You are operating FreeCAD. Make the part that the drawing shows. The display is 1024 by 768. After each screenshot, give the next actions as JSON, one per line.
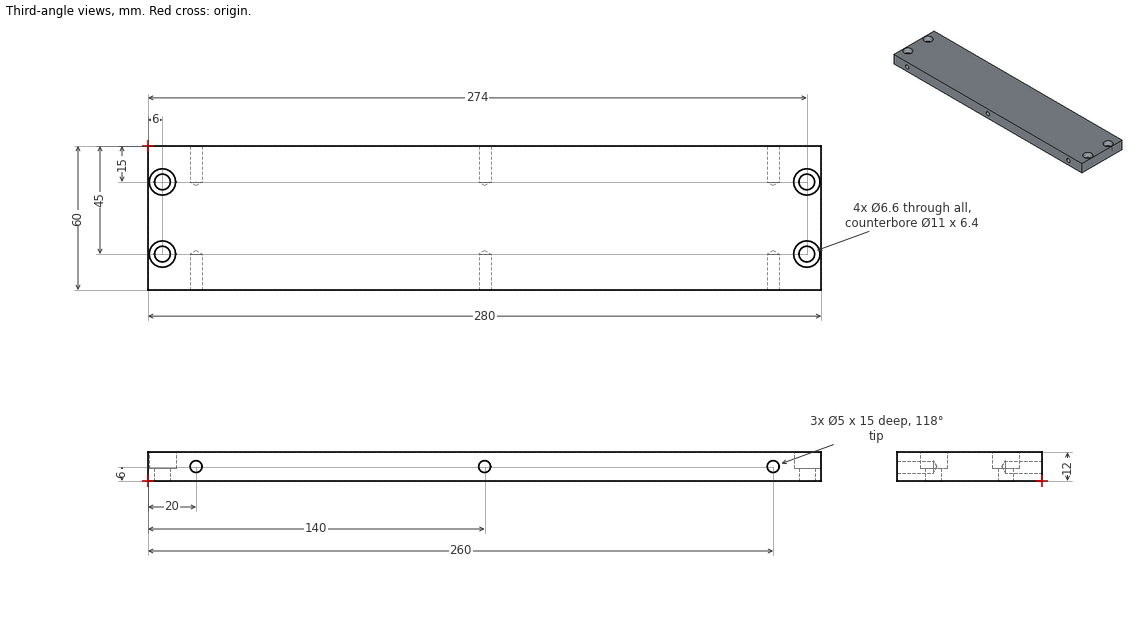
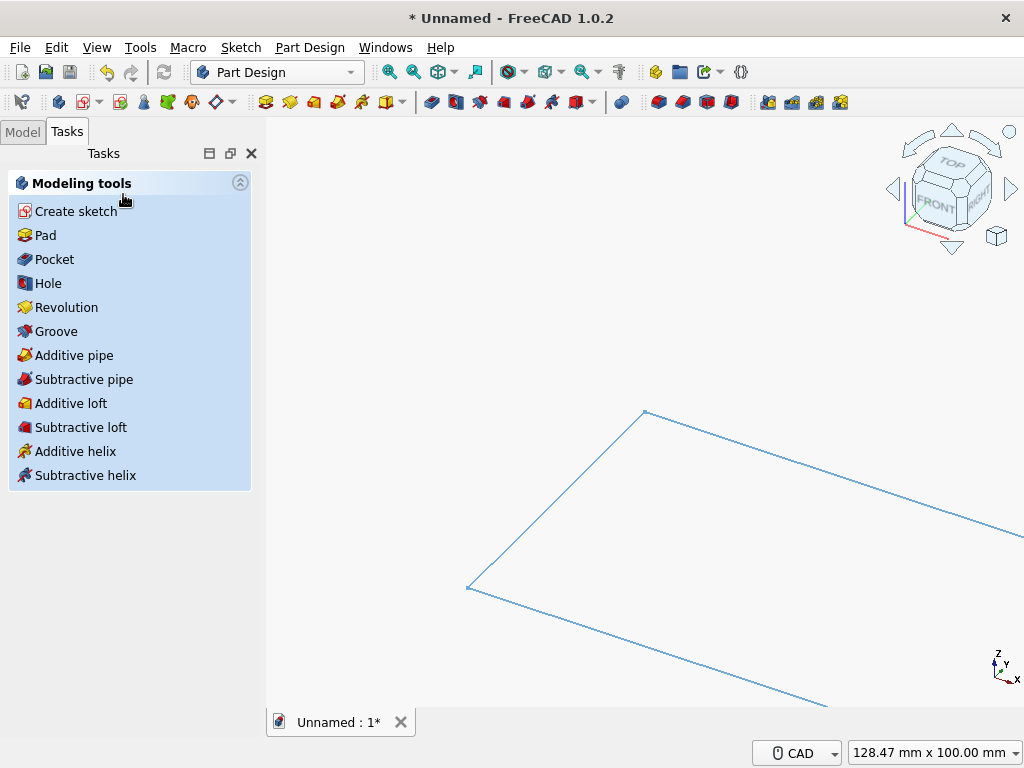
{"action": "left_click", "coordinate": [266, 102]}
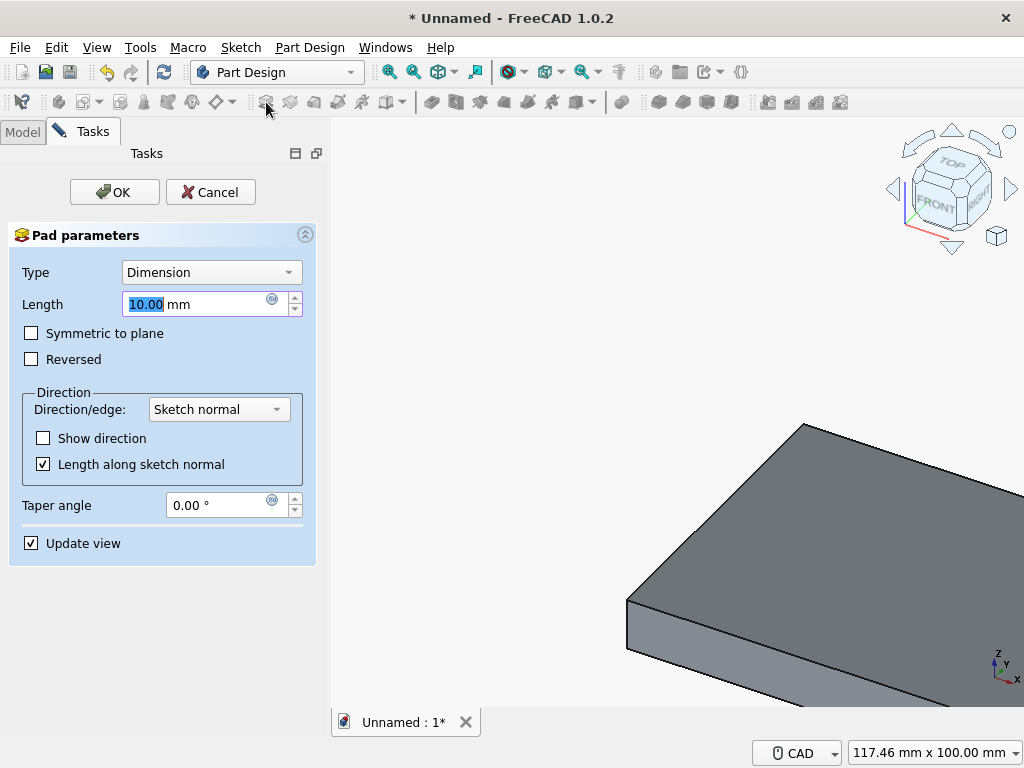
{"action": "type", "text": "12"}
{"action": "key", "text": "Tab"}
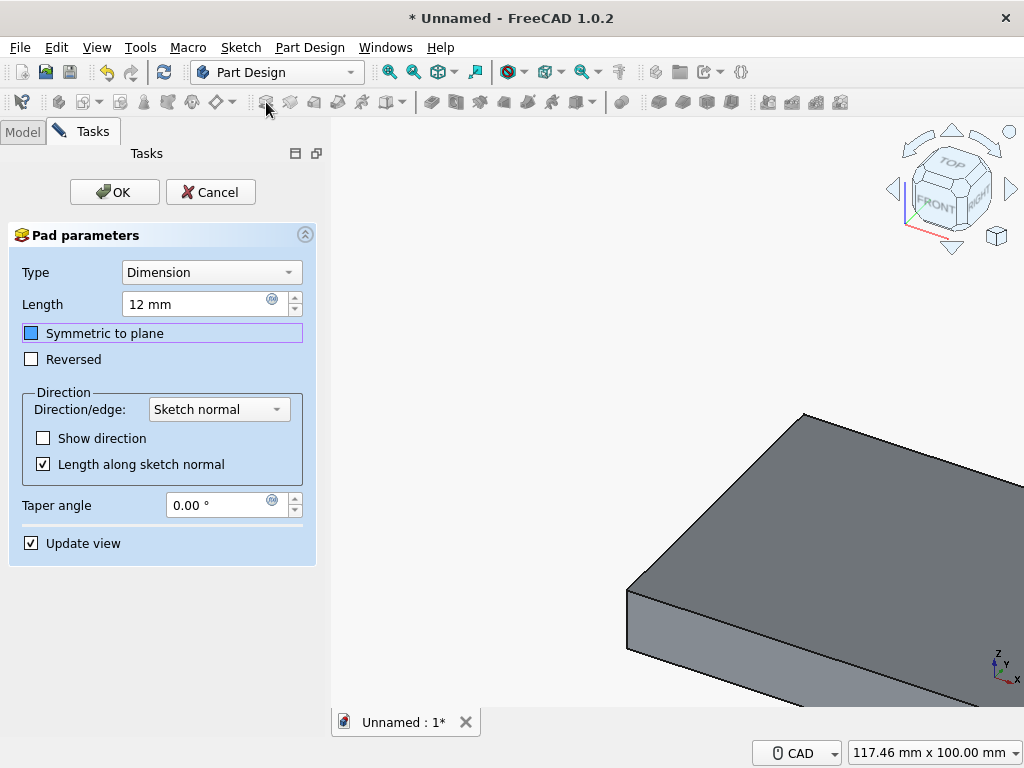
{"action": "left_click", "coordinate": [115, 192]}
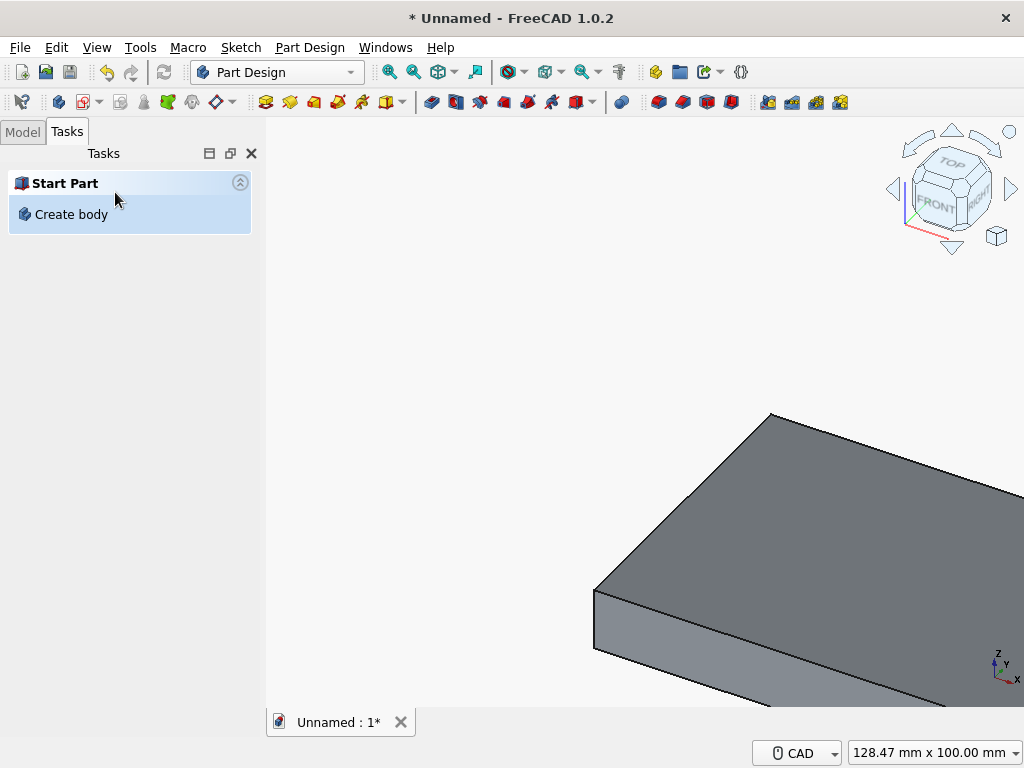
{"action": "left_click", "coordinate": [390, 72]}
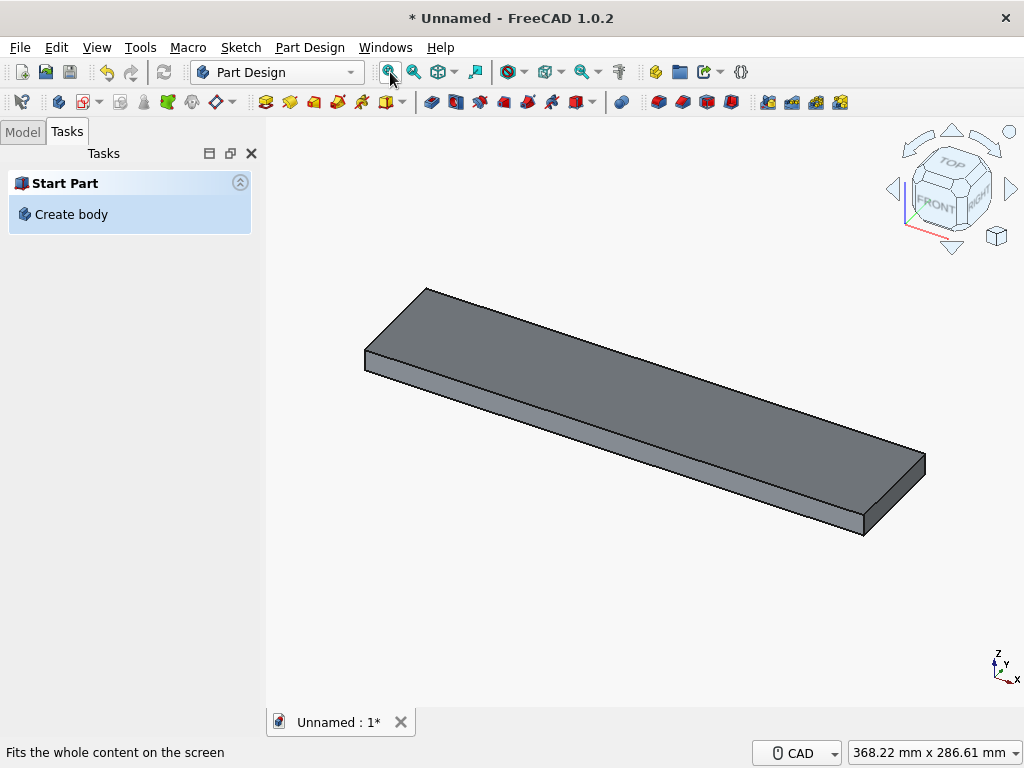
{"action": "left_click", "coordinate": [84, 102]}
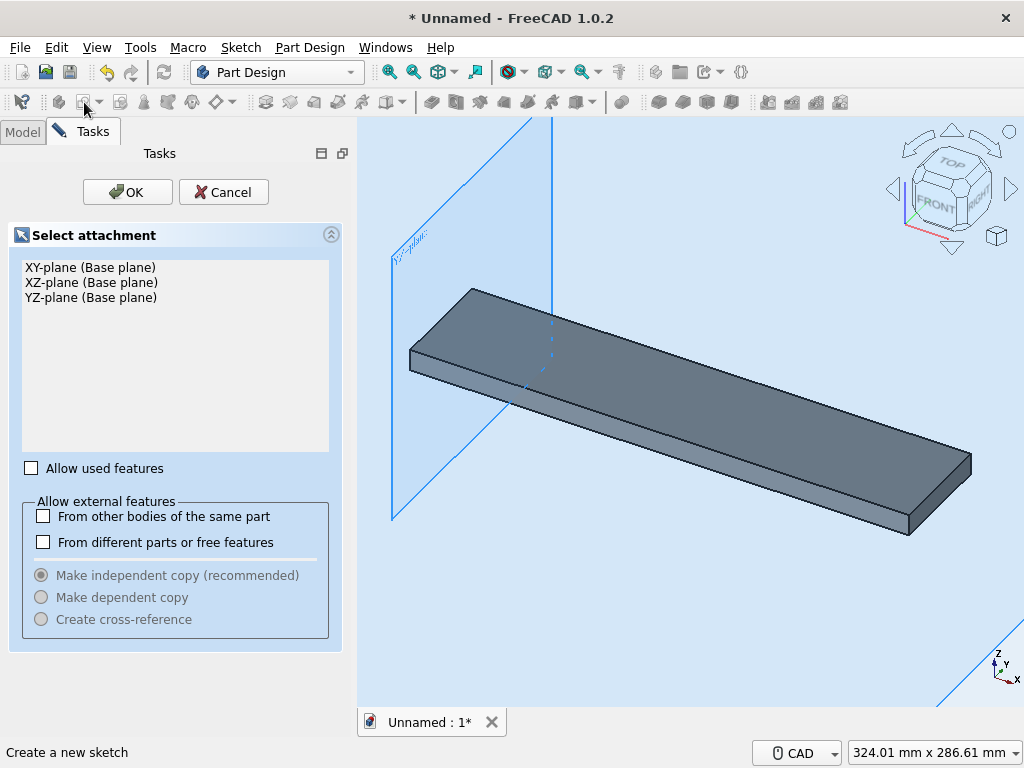
{"action": "left_click", "coordinate": [82, 282]}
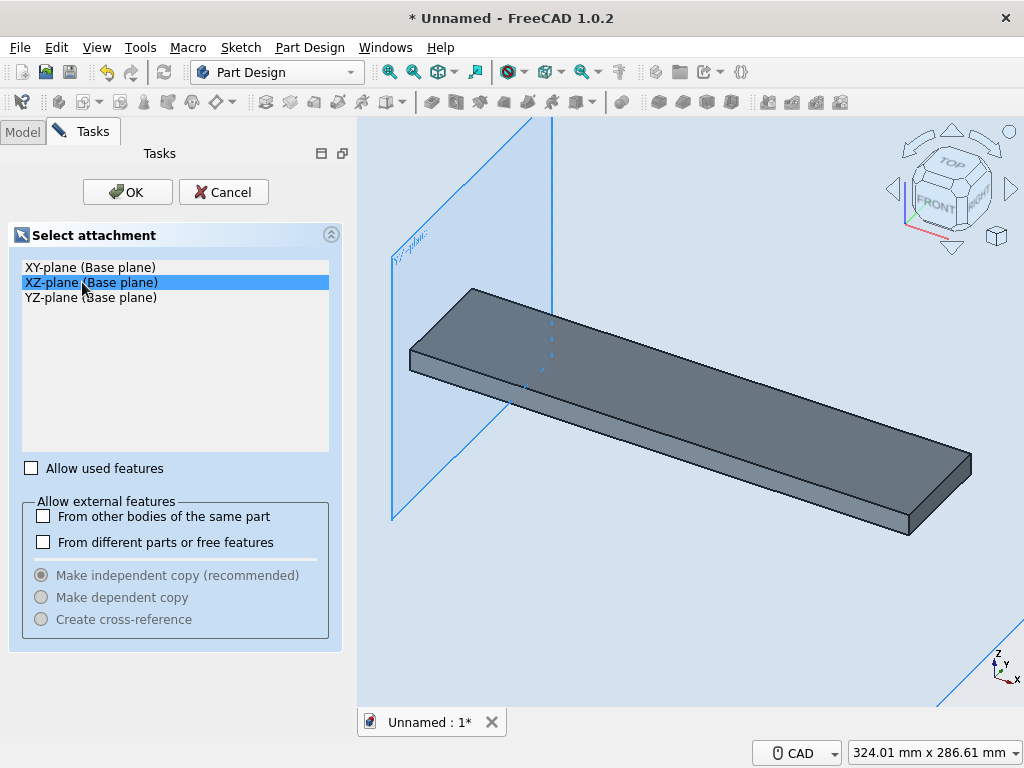
{"action": "left_click", "coordinate": [128, 192]}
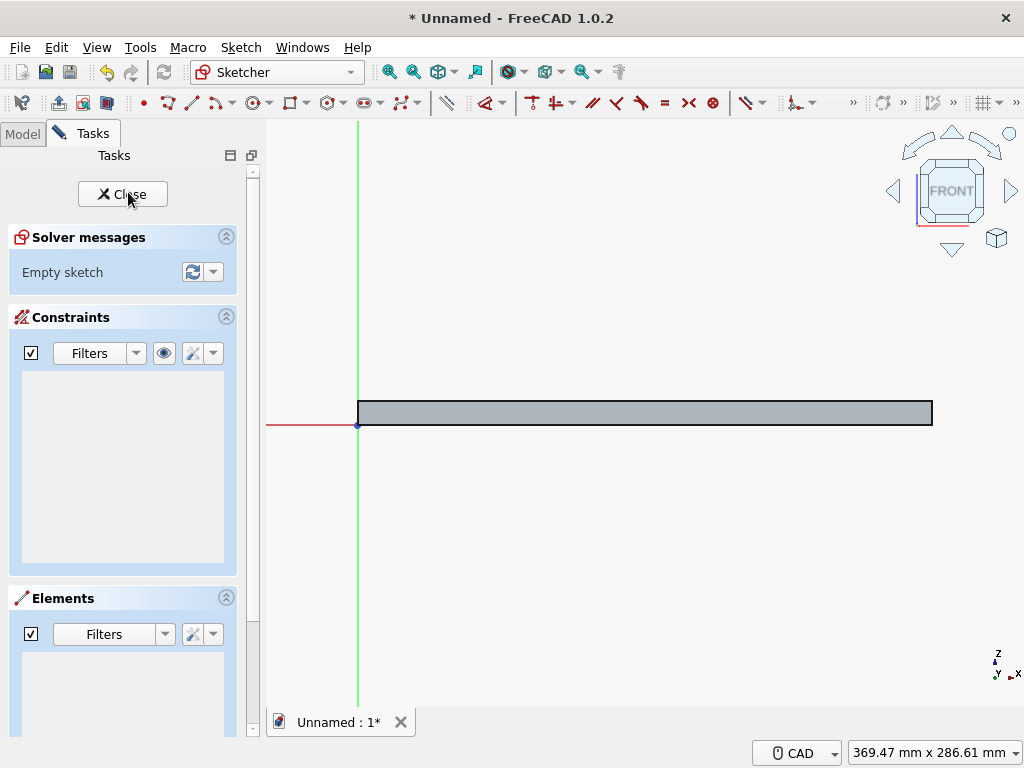
{"action": "left_click", "coordinate": [108, 104]}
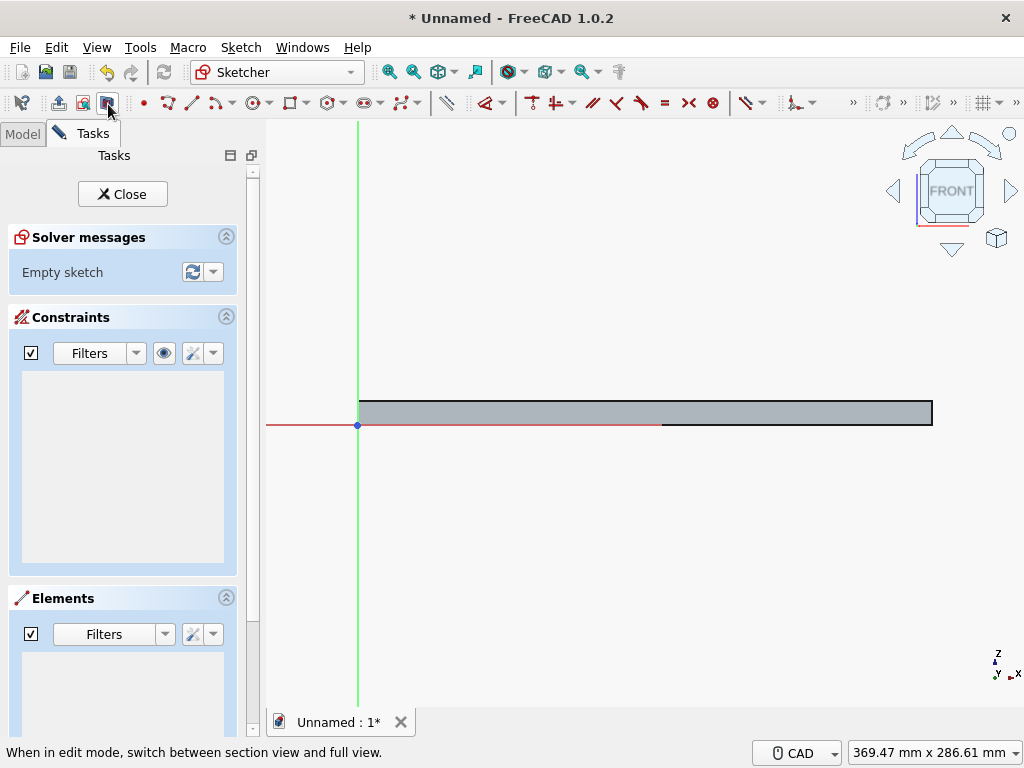
{"action": "scroll", "coordinate": [474, 406], "scroll_direction": "down", "scroll_amount": 2}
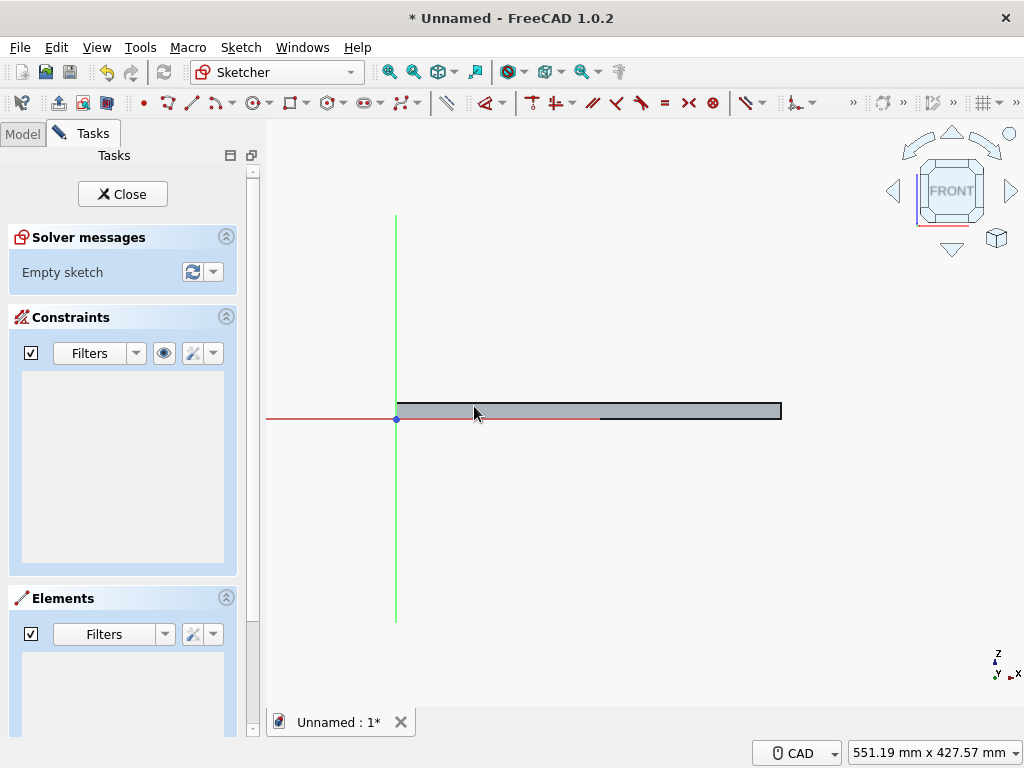
{"action": "left_click", "coordinate": [254, 104]}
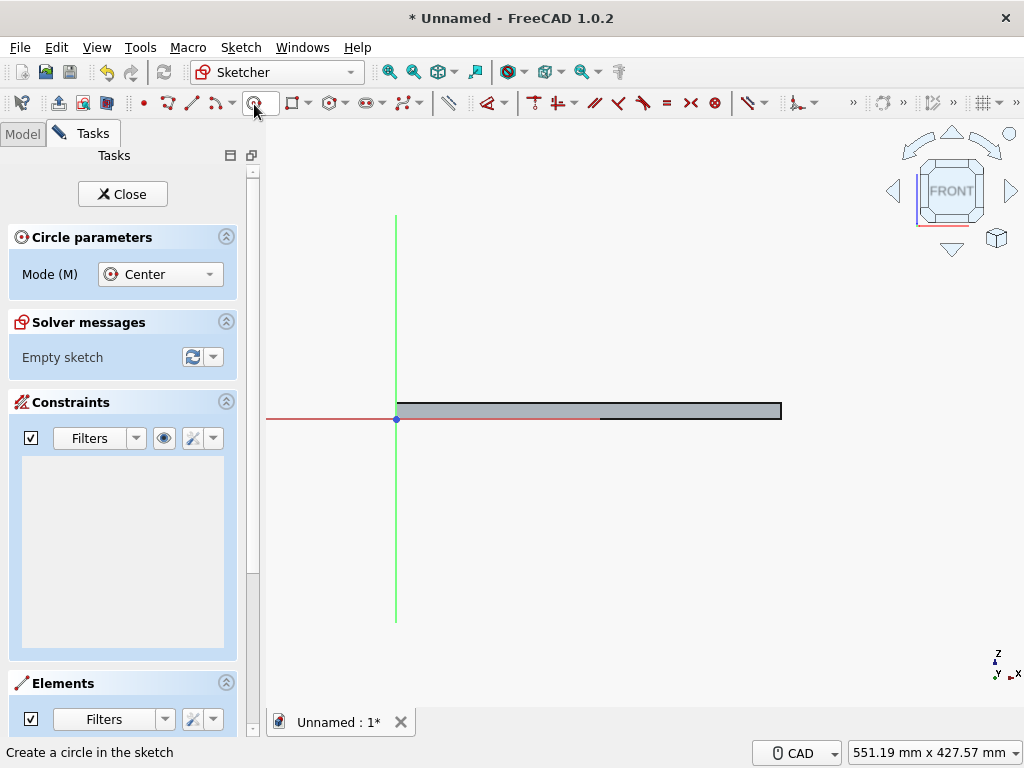
{"action": "scroll", "coordinate": [754, 411], "scroll_direction": "up", "scroll_amount": 10}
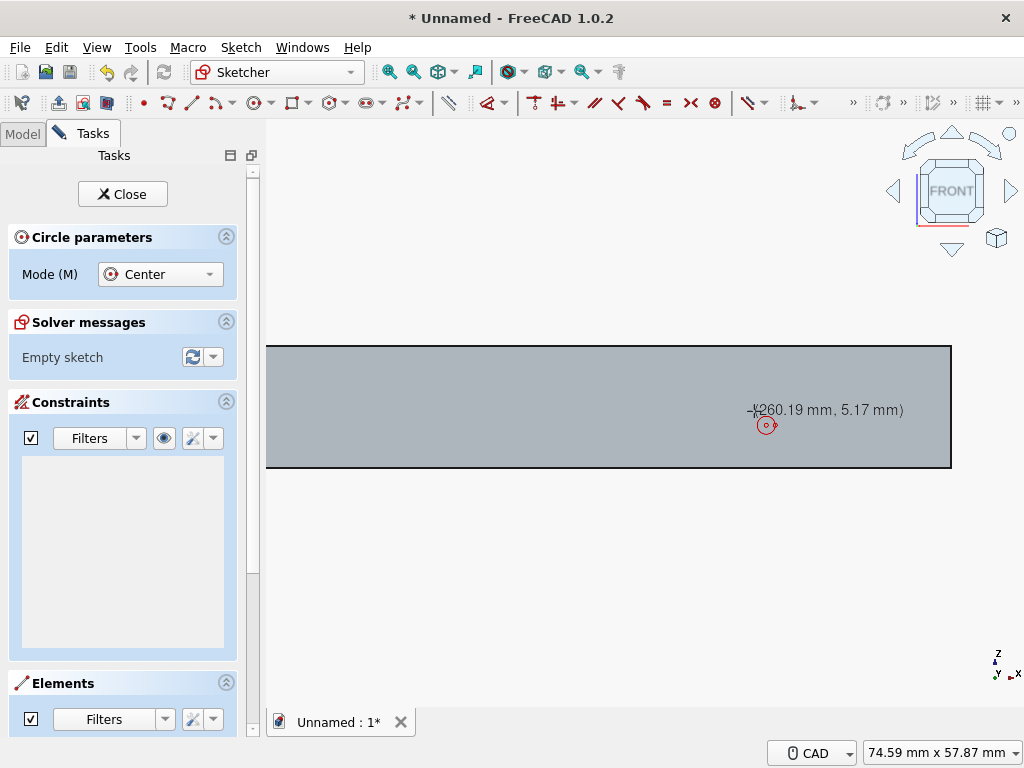
{"action": "scroll", "coordinate": [754, 411], "scroll_direction": "down", "scroll_amount": 10}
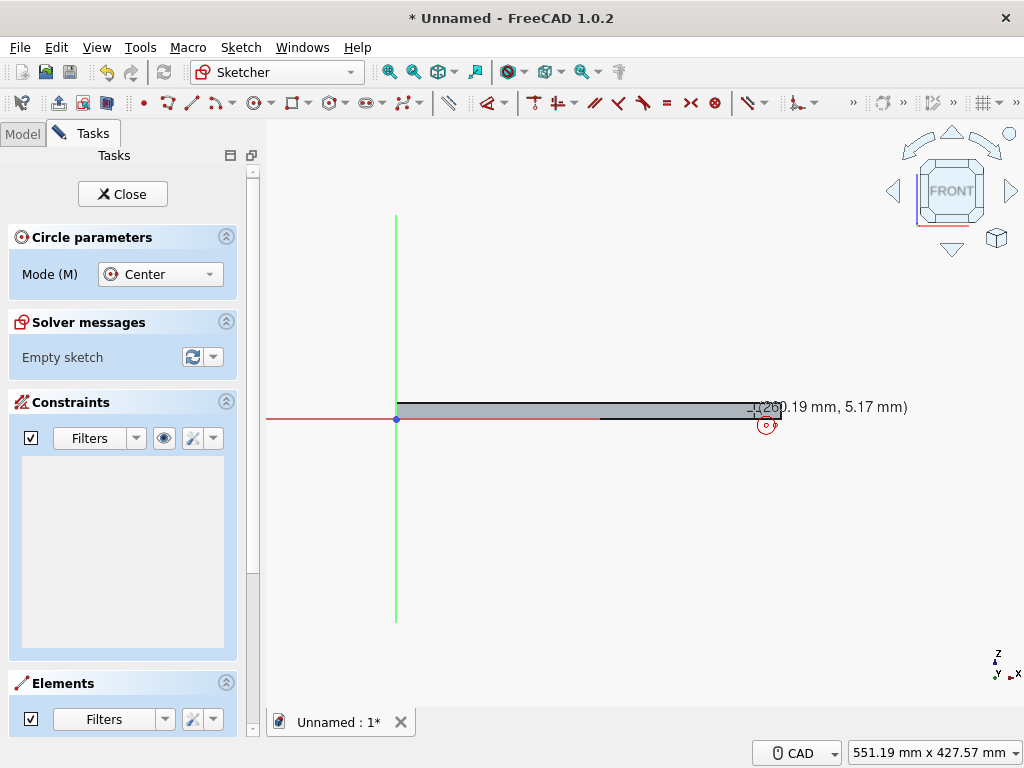
{"action": "scroll", "coordinate": [754, 411], "scroll_direction": "up", "scroll_amount": 4}